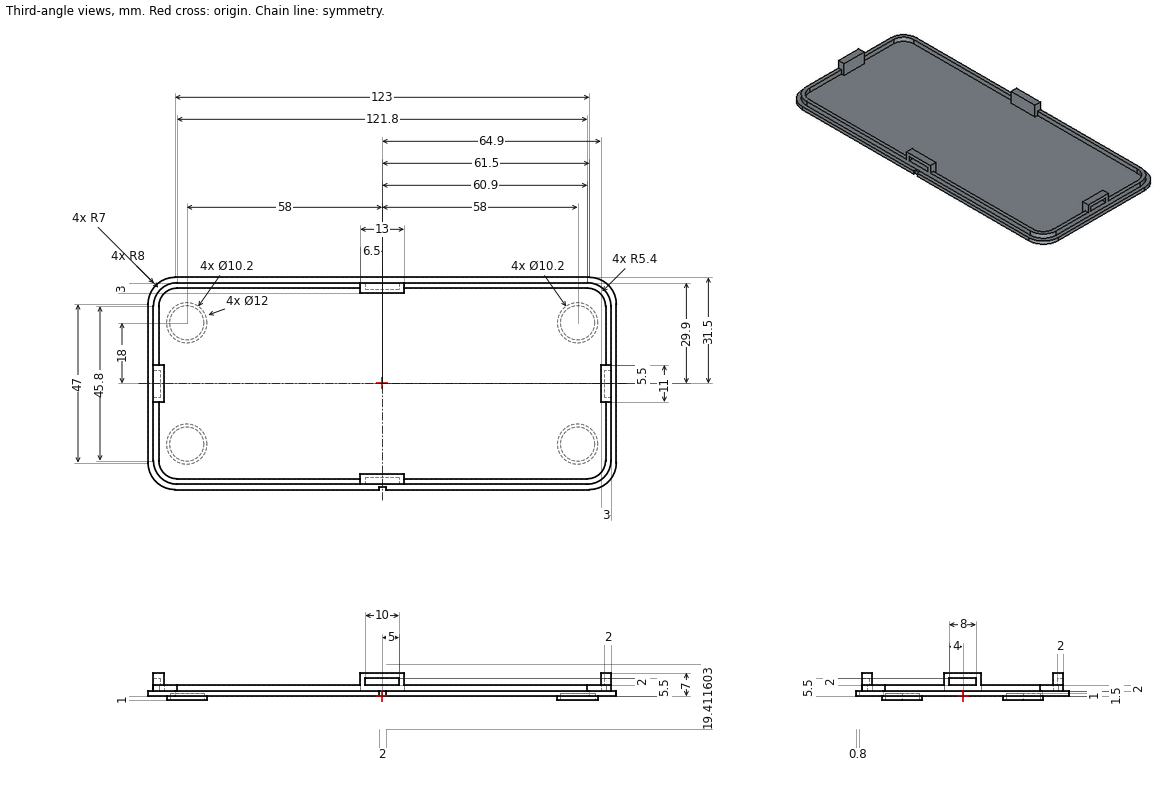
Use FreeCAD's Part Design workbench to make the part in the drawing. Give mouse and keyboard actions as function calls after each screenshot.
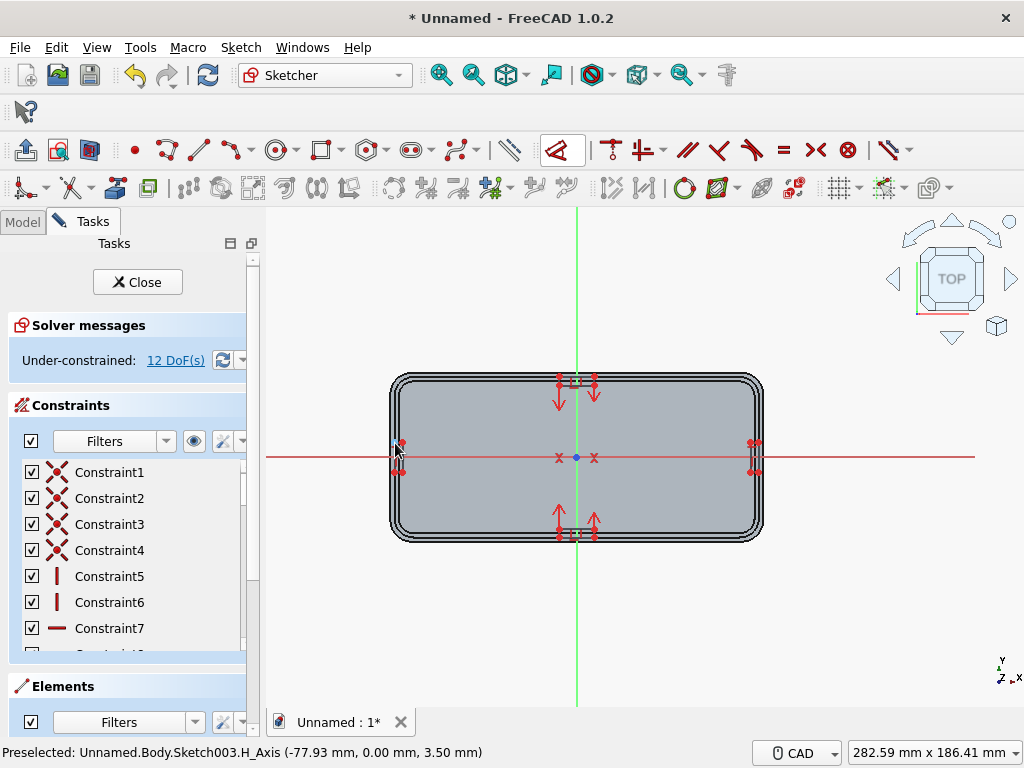
scroll(759, 443, up, 3)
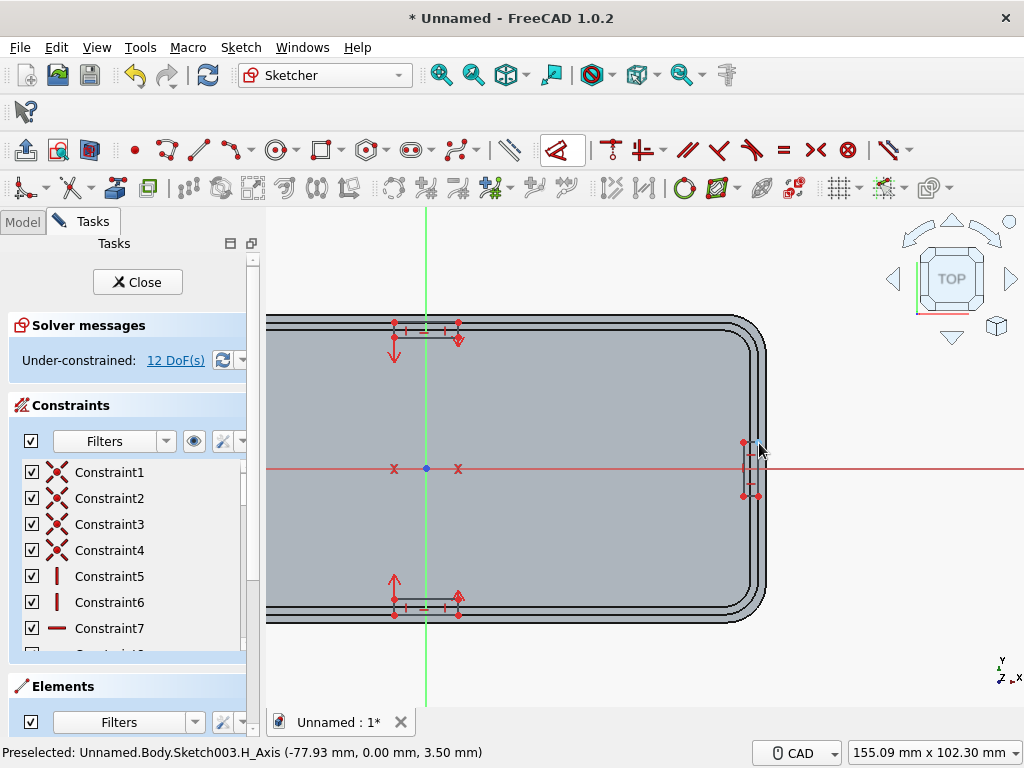
click(758, 442)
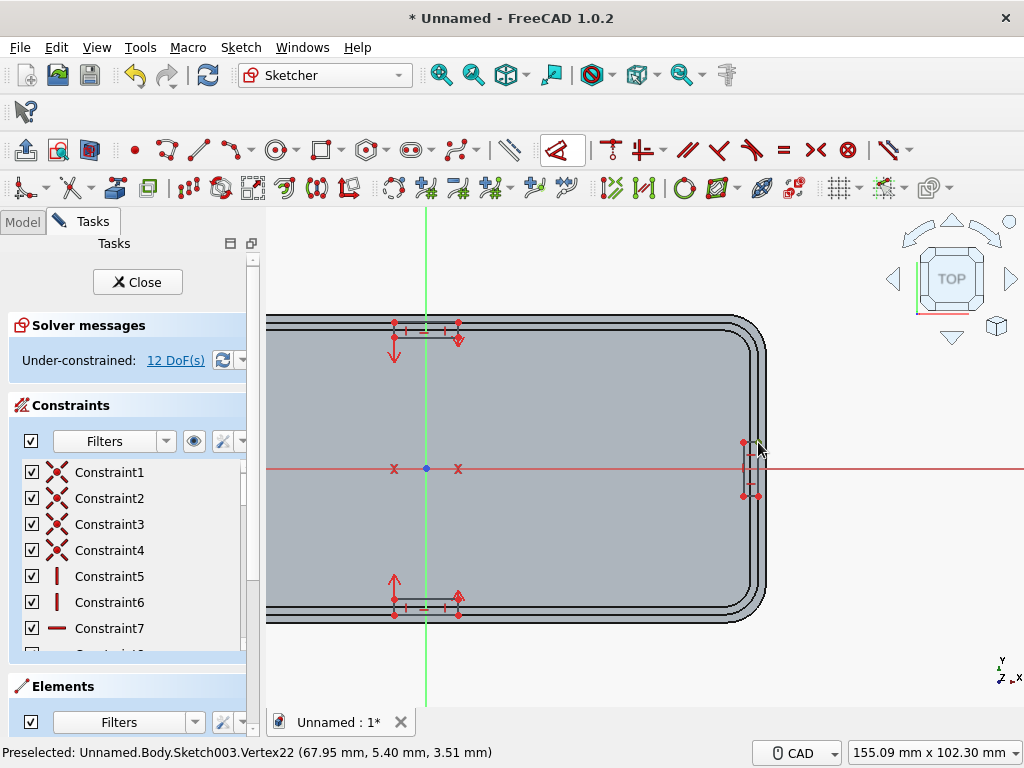
scroll(759, 443, down, 3)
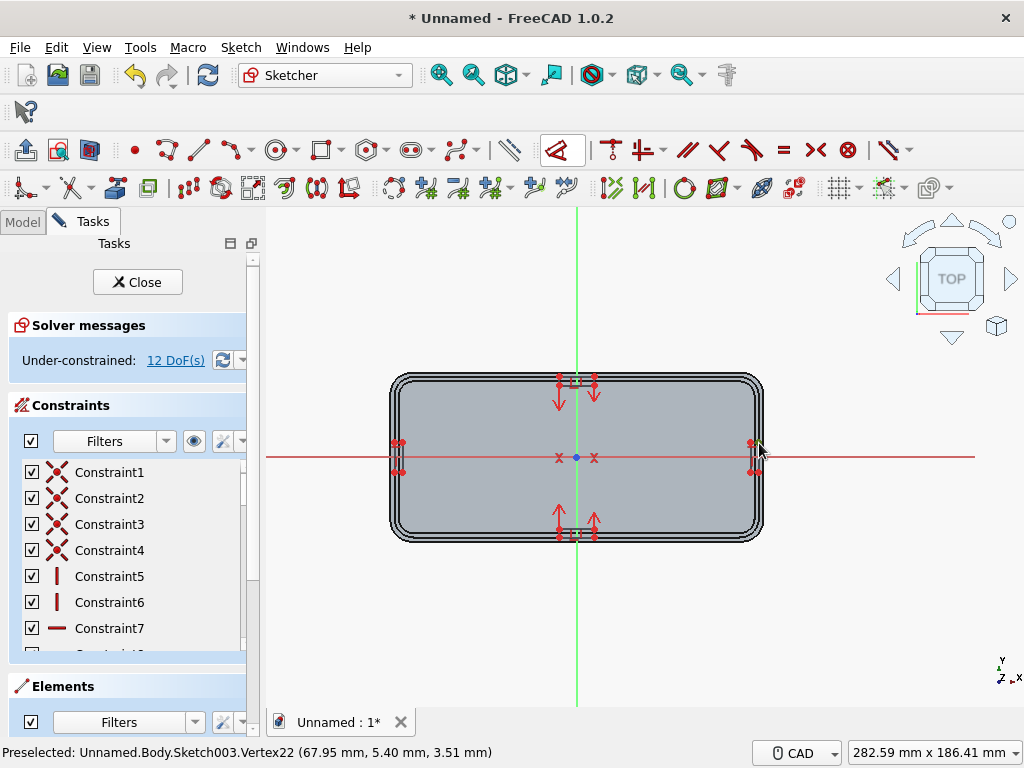
scroll(395, 443, up, 3)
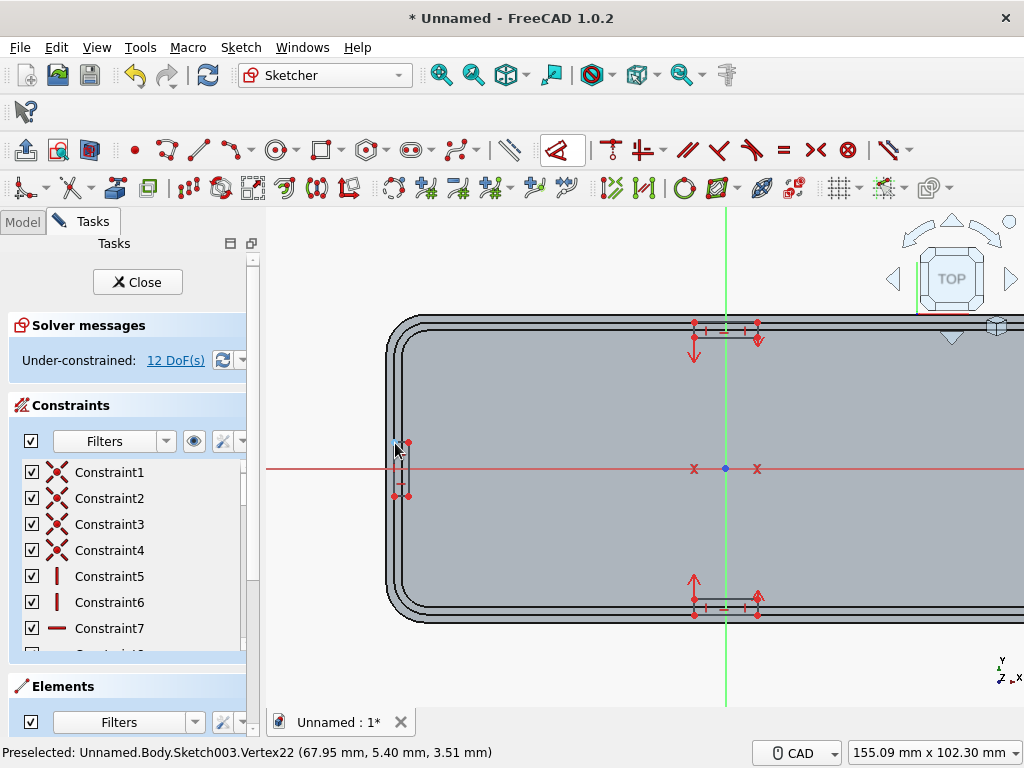
click(394, 442)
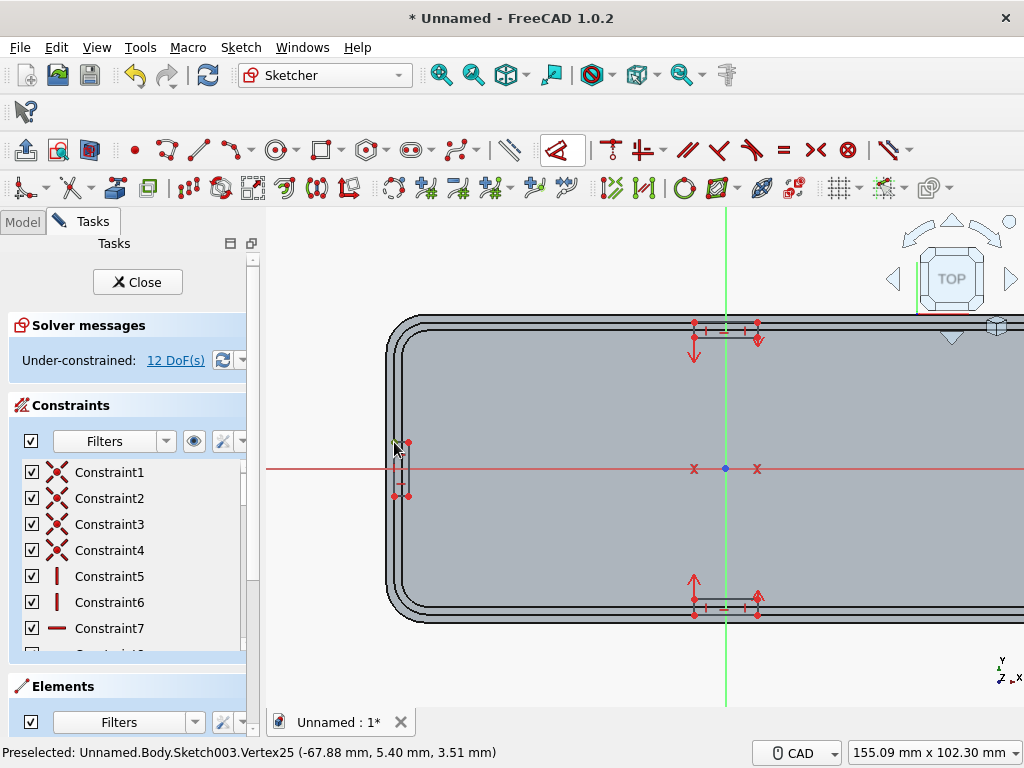
click(726, 647)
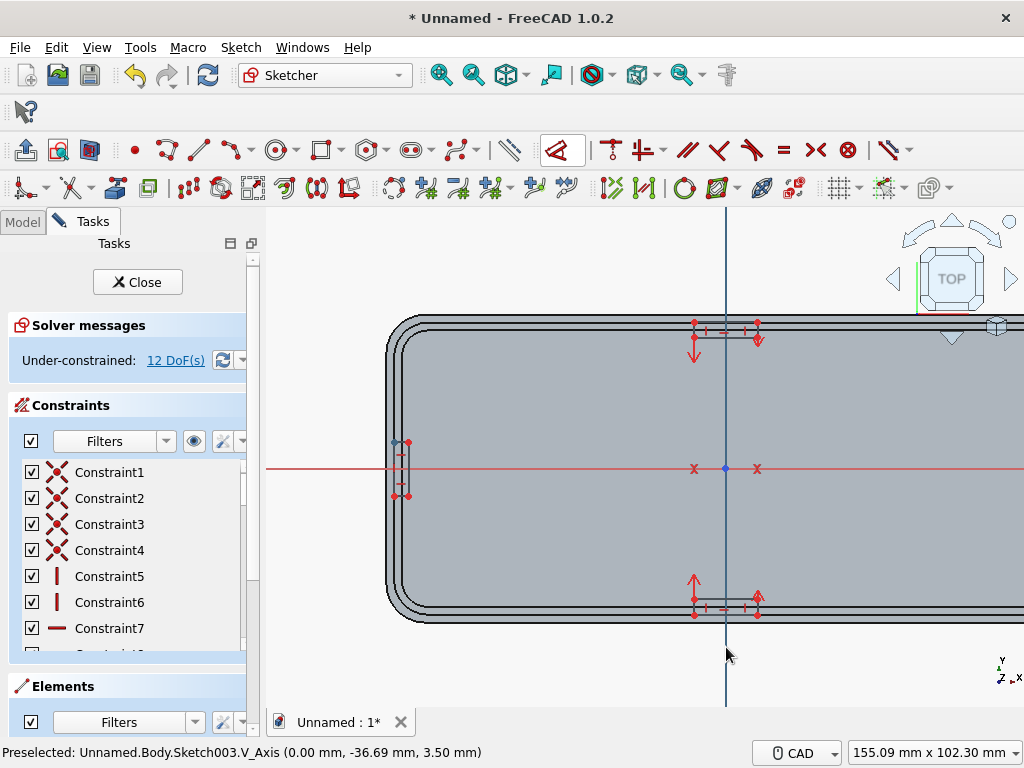
key(s)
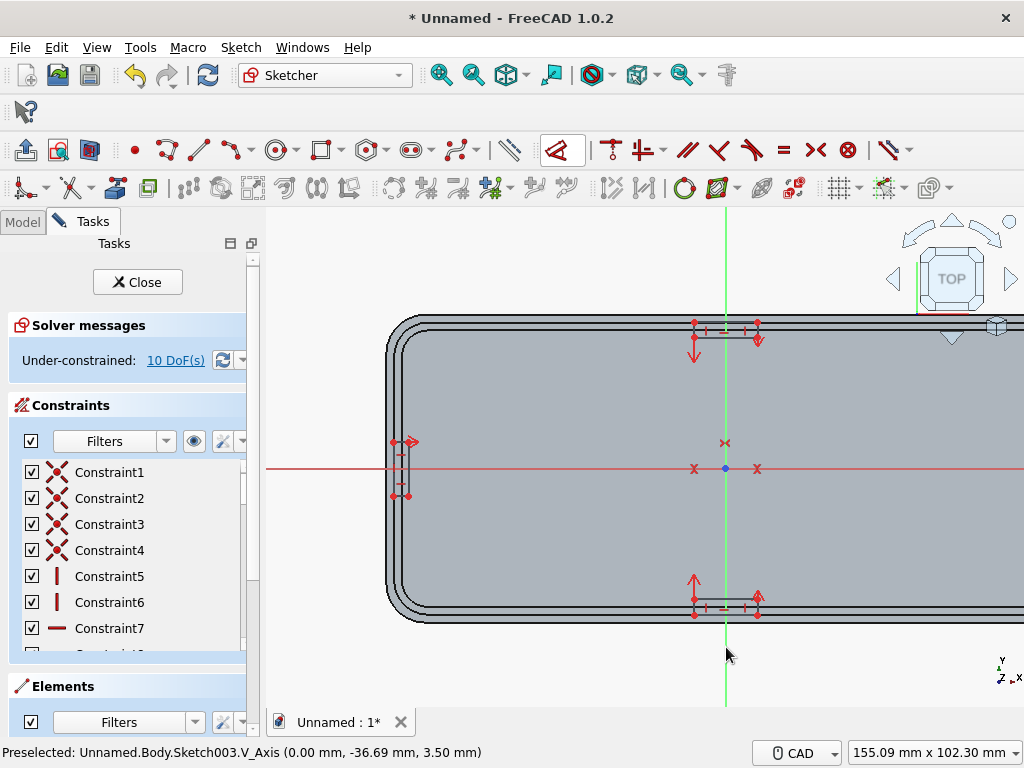
scroll(395, 443, down, 3)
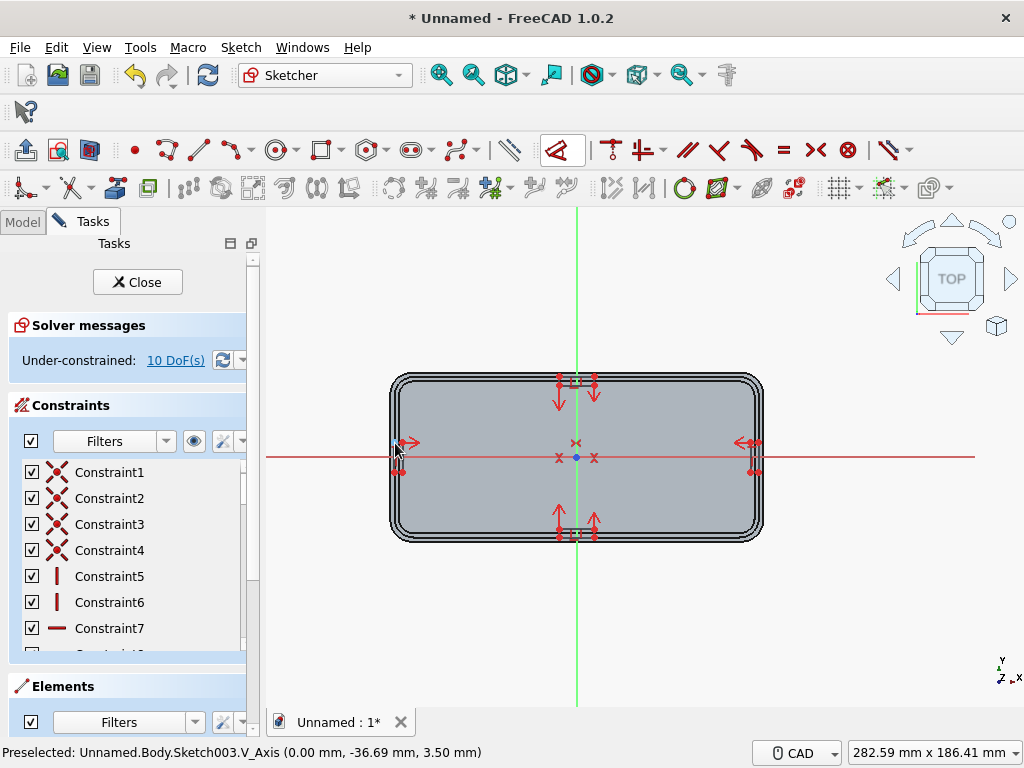
scroll(751, 472, up, 3)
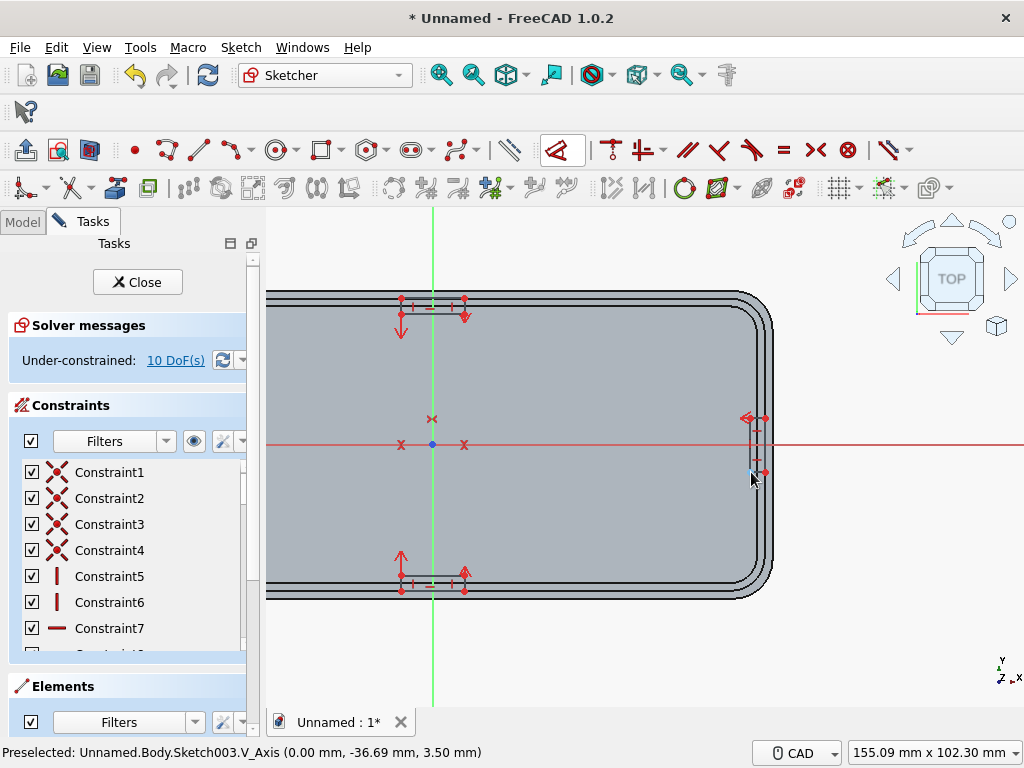
click(750, 472)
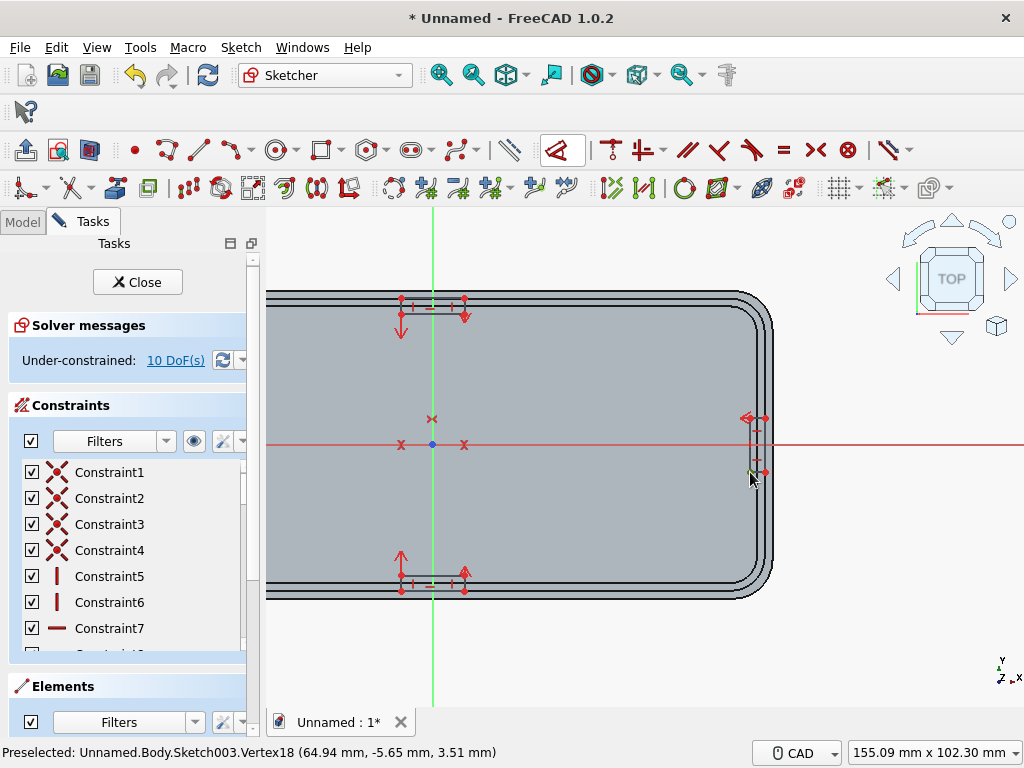
scroll(751, 472, down, 3)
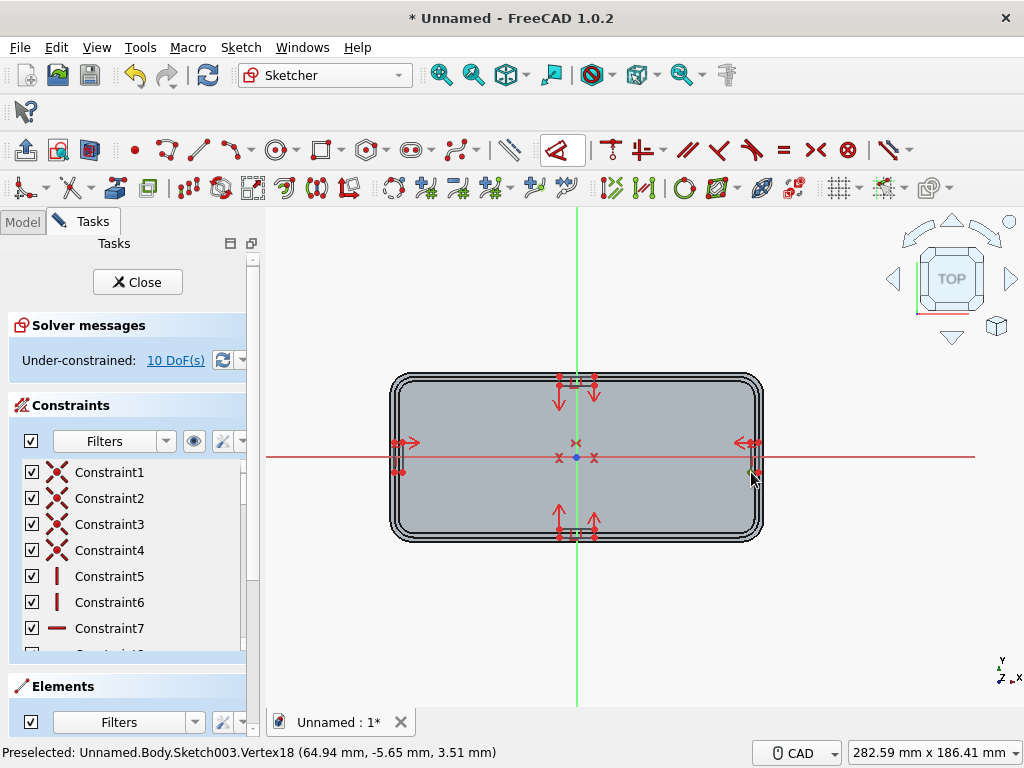
scroll(403, 472, up, 2)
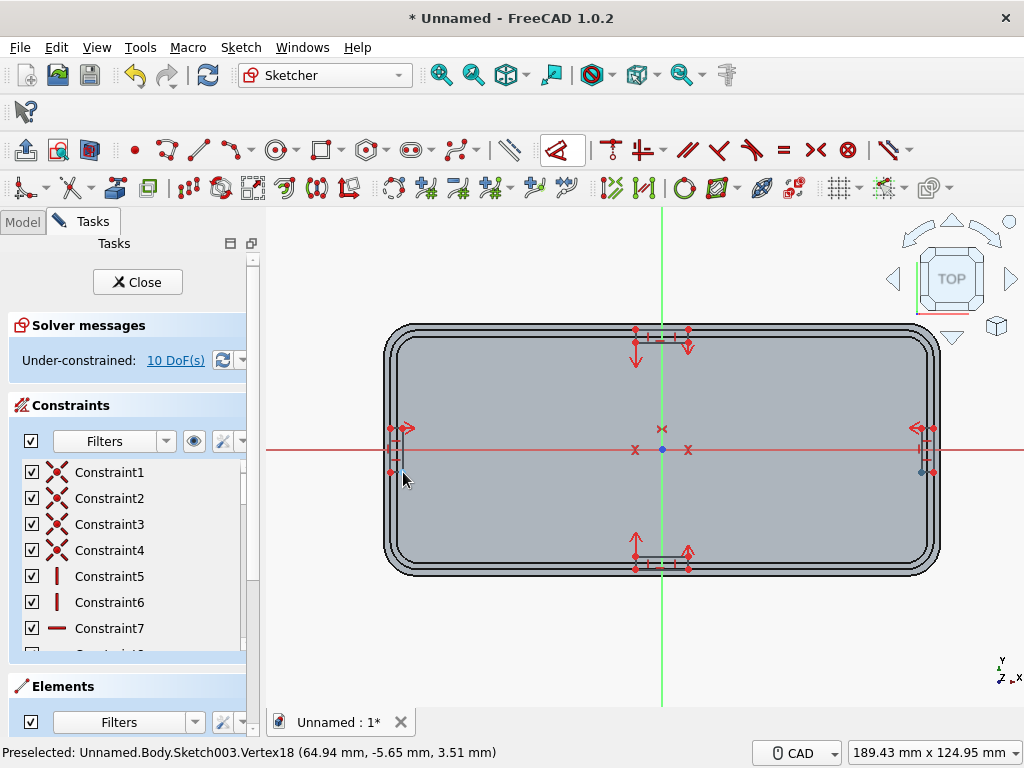
click(403, 472)